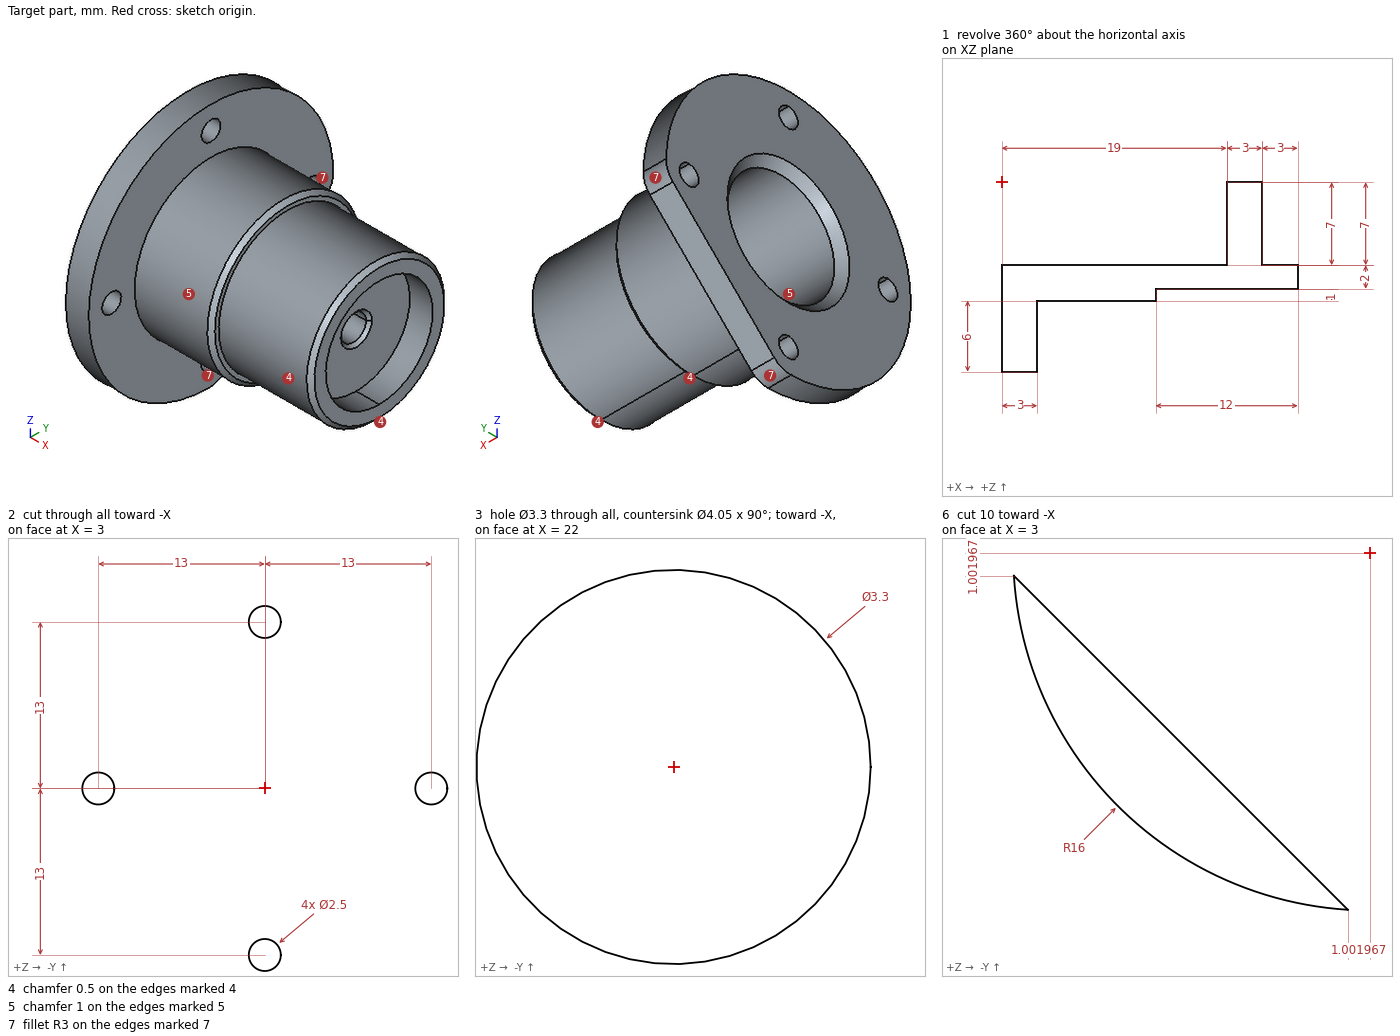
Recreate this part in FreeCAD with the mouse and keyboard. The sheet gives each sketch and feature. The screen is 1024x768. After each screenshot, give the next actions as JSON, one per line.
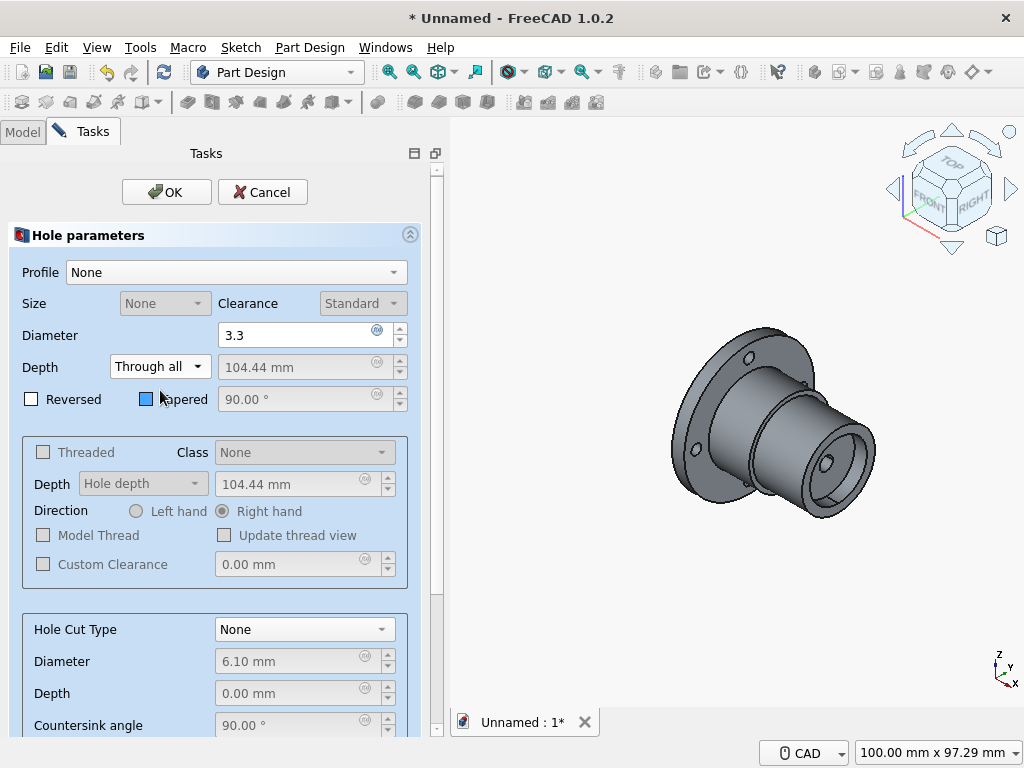
{"action": "left_click", "coordinate": [306, 630]}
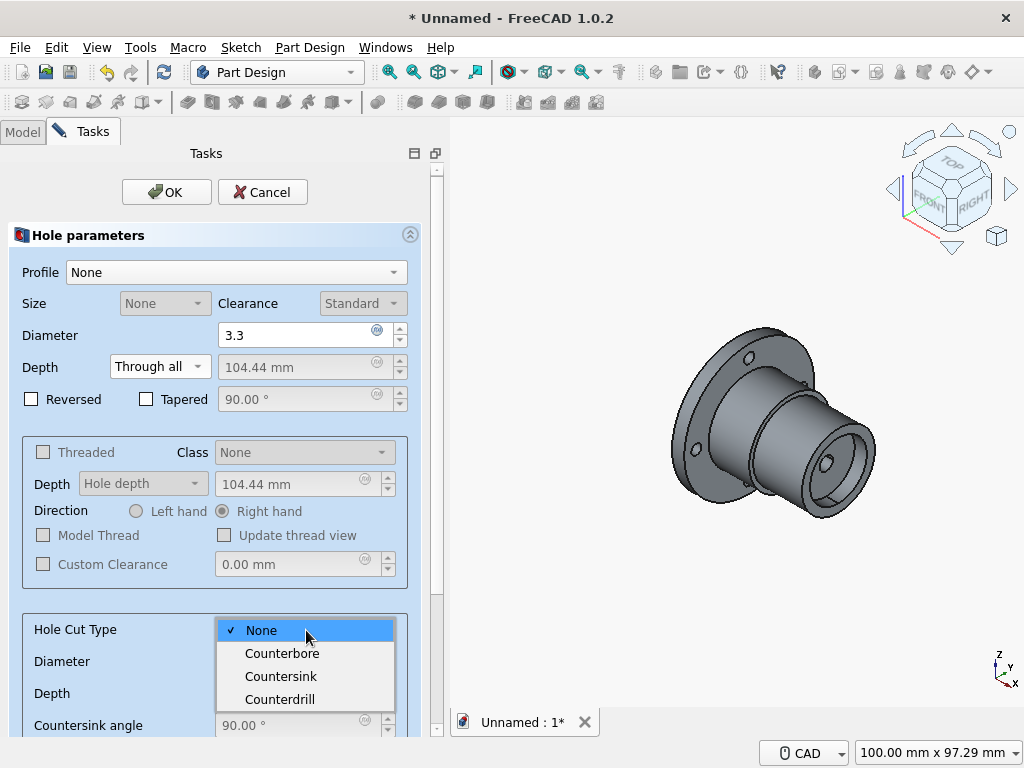
{"action": "left_click", "coordinate": [304, 676]}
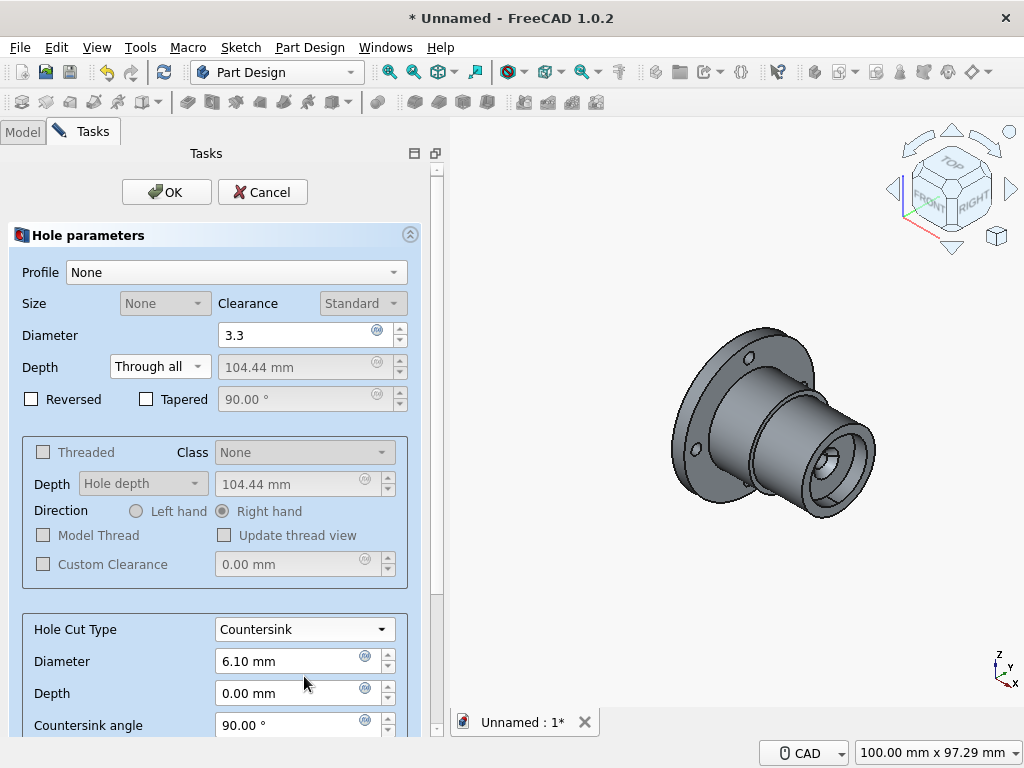
{"action": "triple_click", "coordinate": [298, 661]}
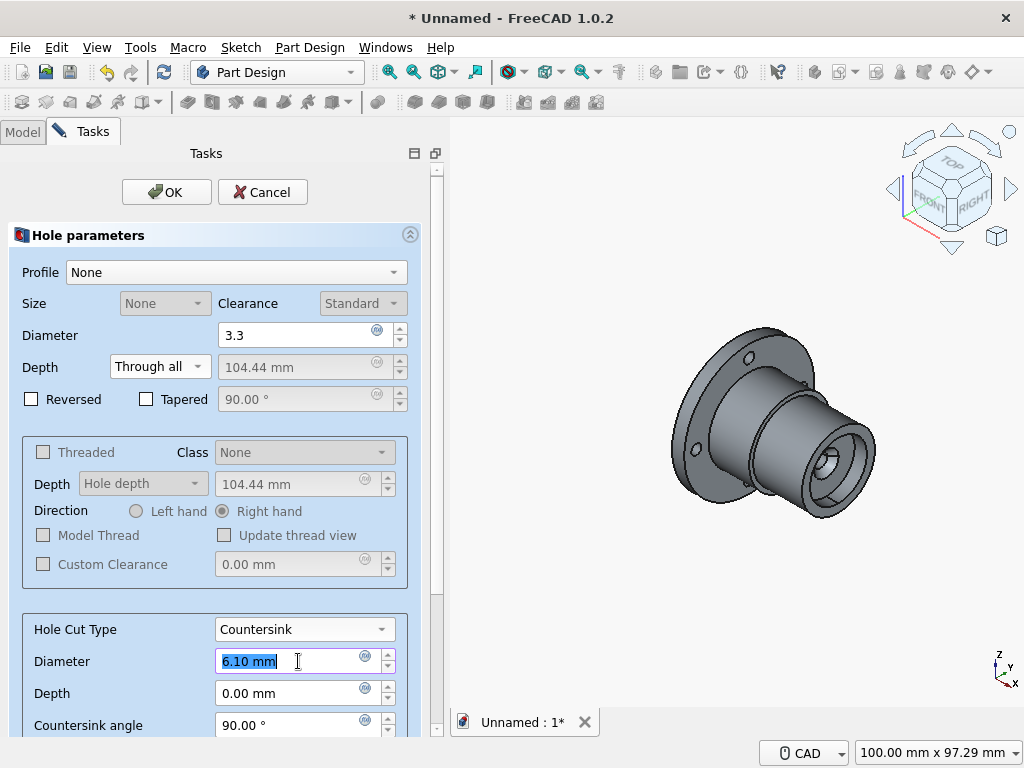
{"action": "type", "text": "4.05"}
{"action": "key", "text": "Tab"}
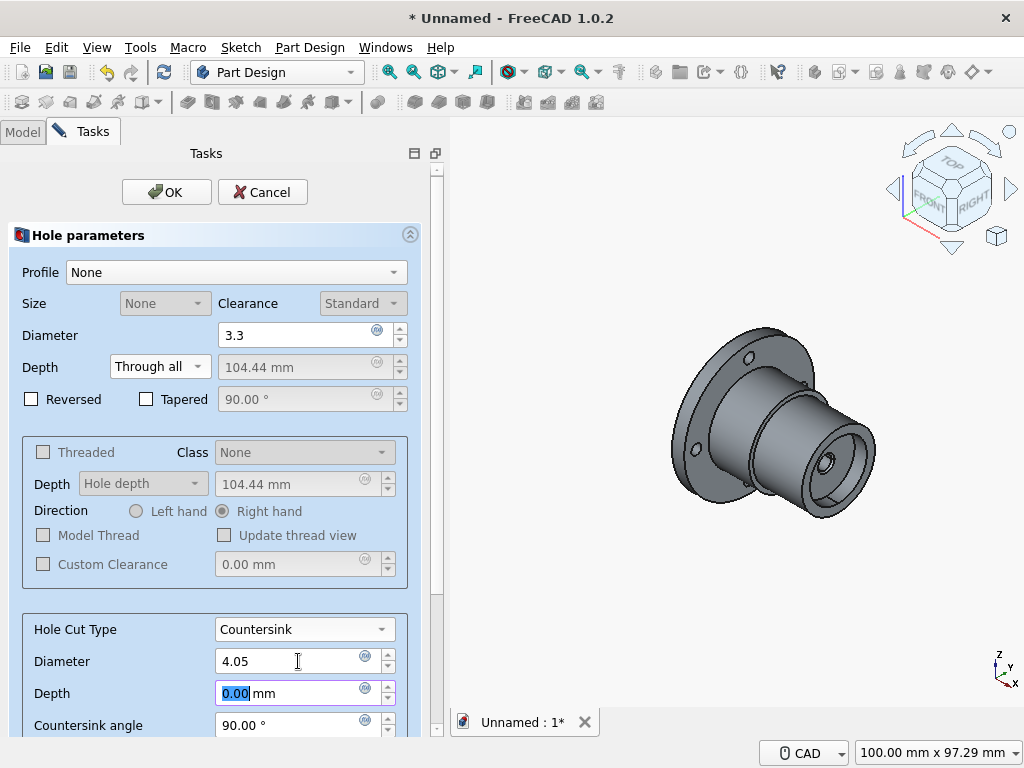
{"action": "left_click", "coordinate": [167, 192]}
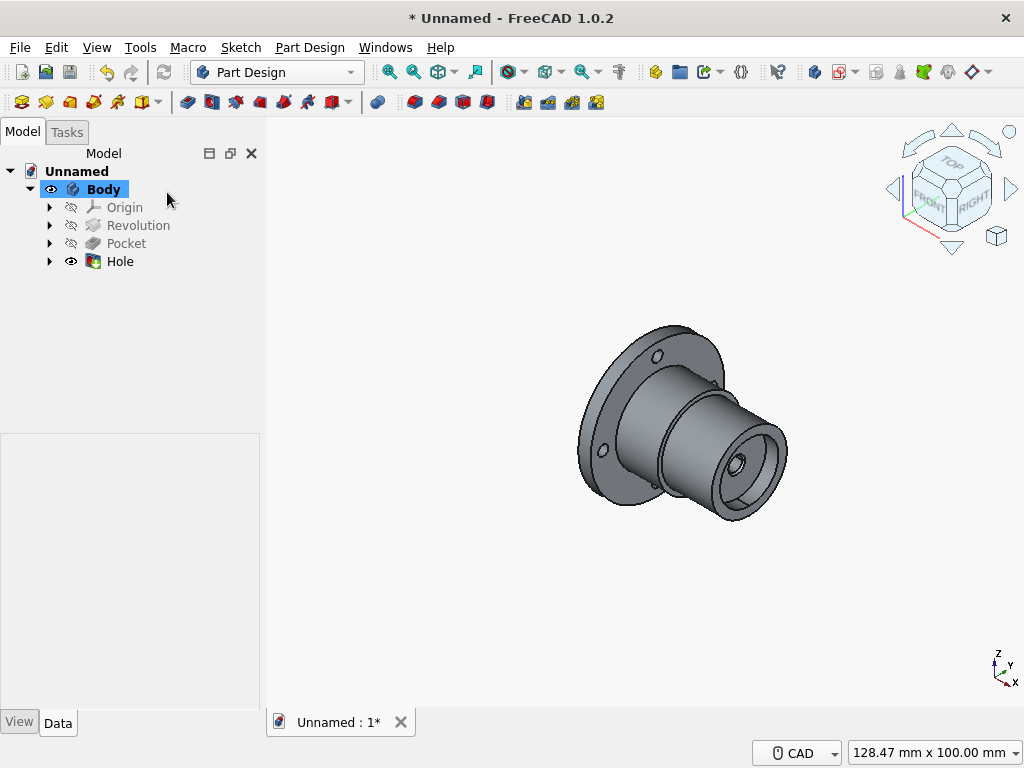
{"action": "left_click", "coordinate": [749, 428]}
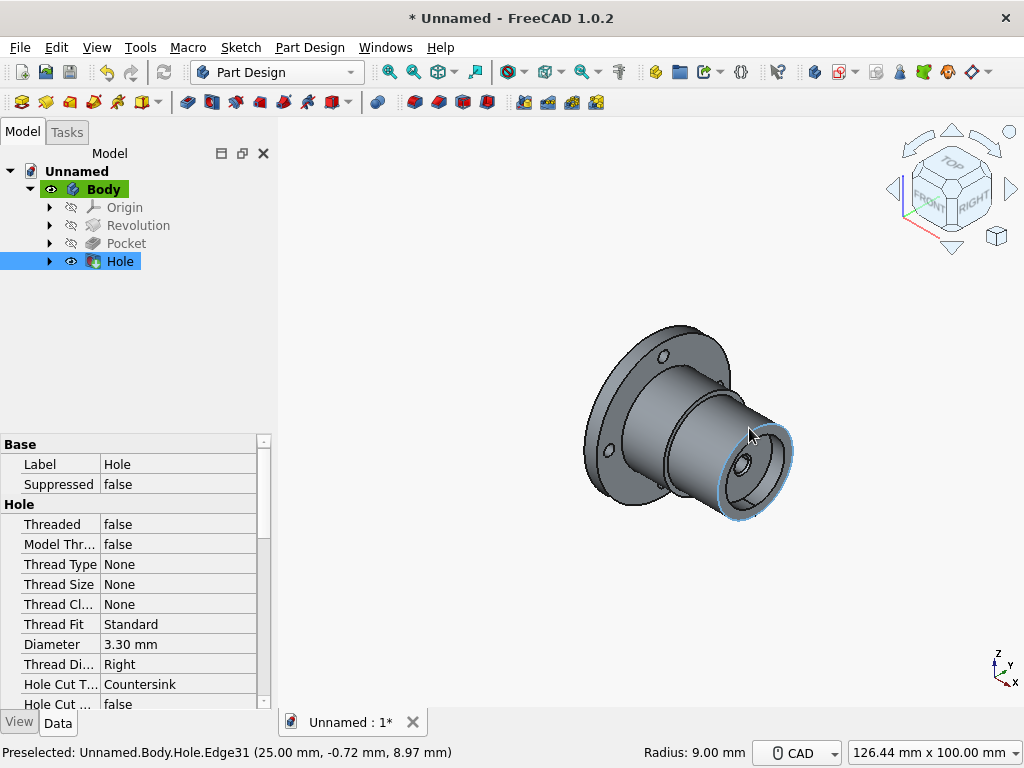
{"action": "left_click", "coordinate": [705, 394], "text": "ctrl"}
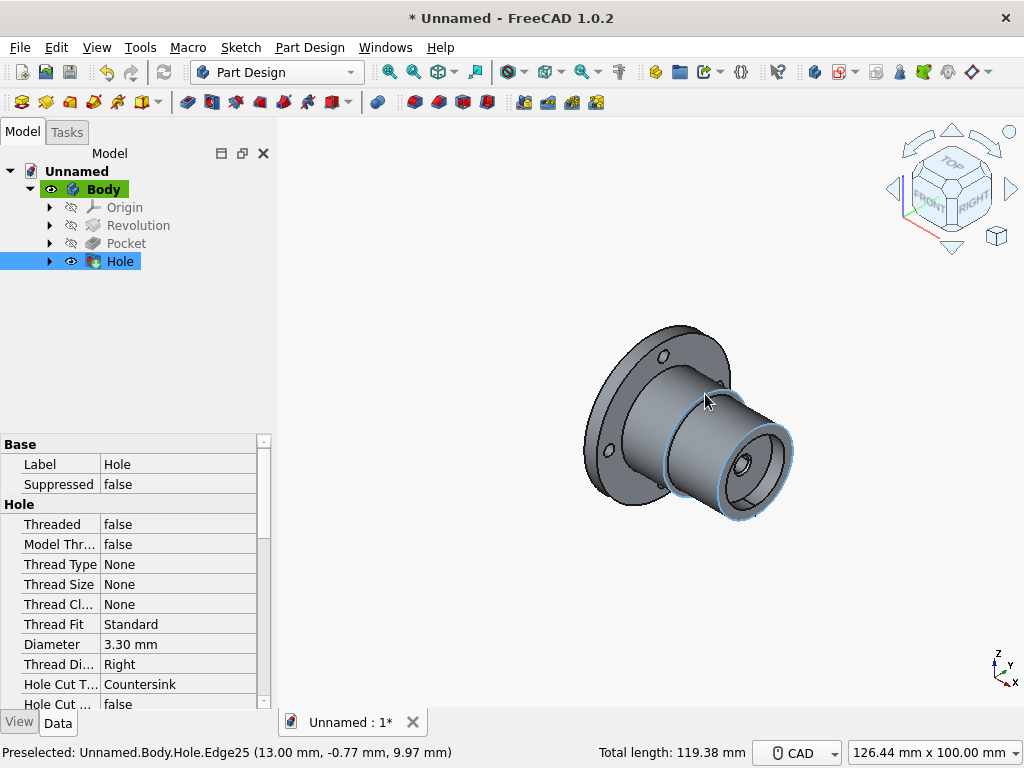
{"action": "left_click", "coordinate": [440, 102]}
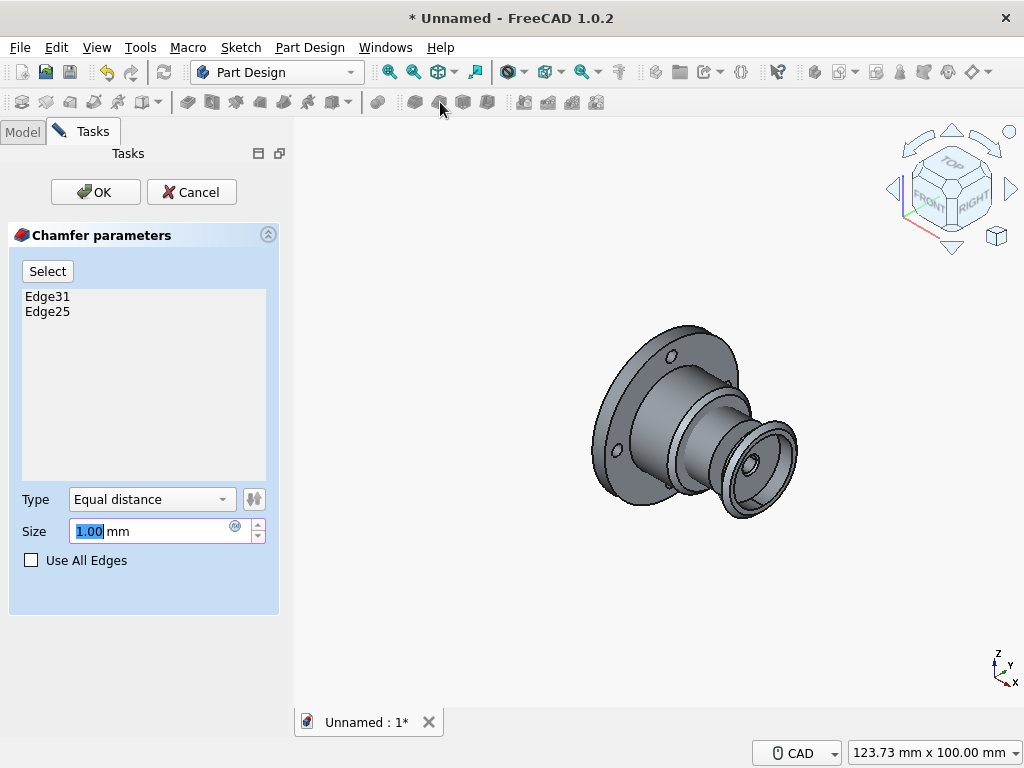
{"action": "type", "text": "0.5"}
{"action": "key", "text": "Tab"}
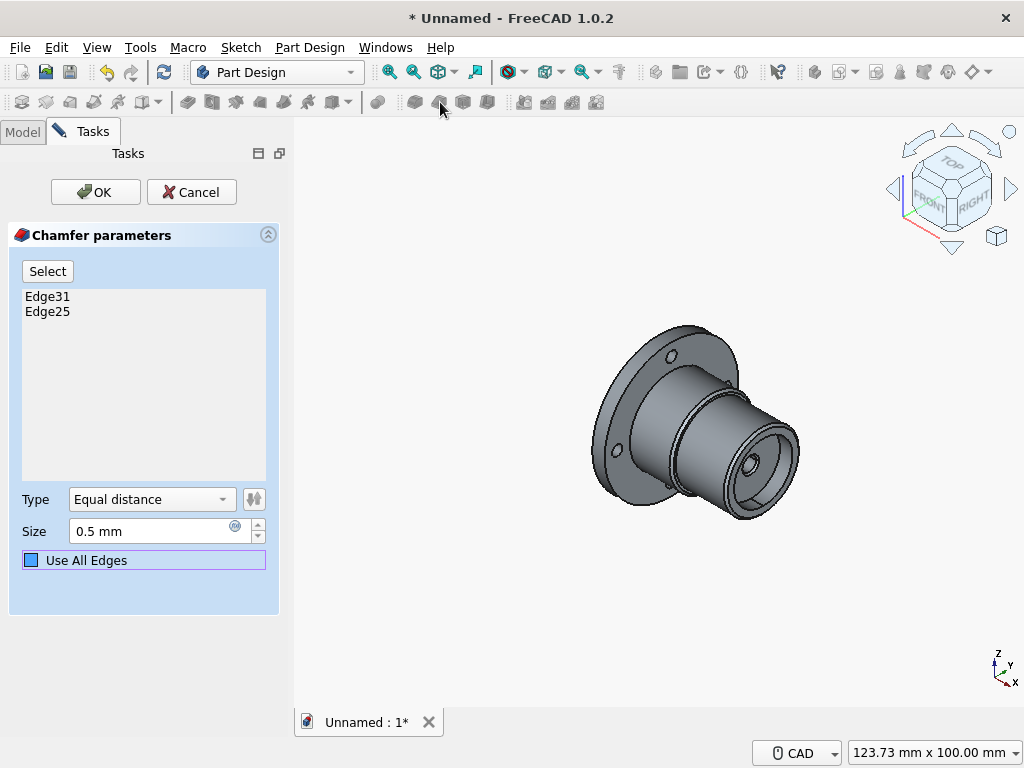
{"action": "left_click", "coordinate": [96, 192]}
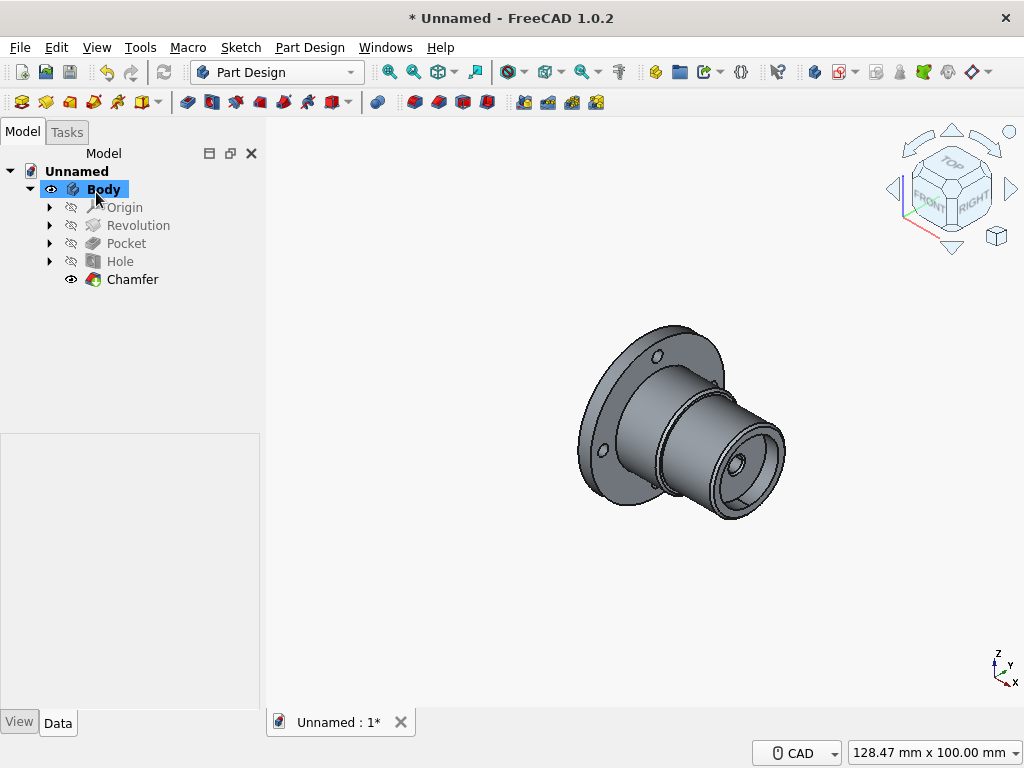
{"action": "key", "text": "2"}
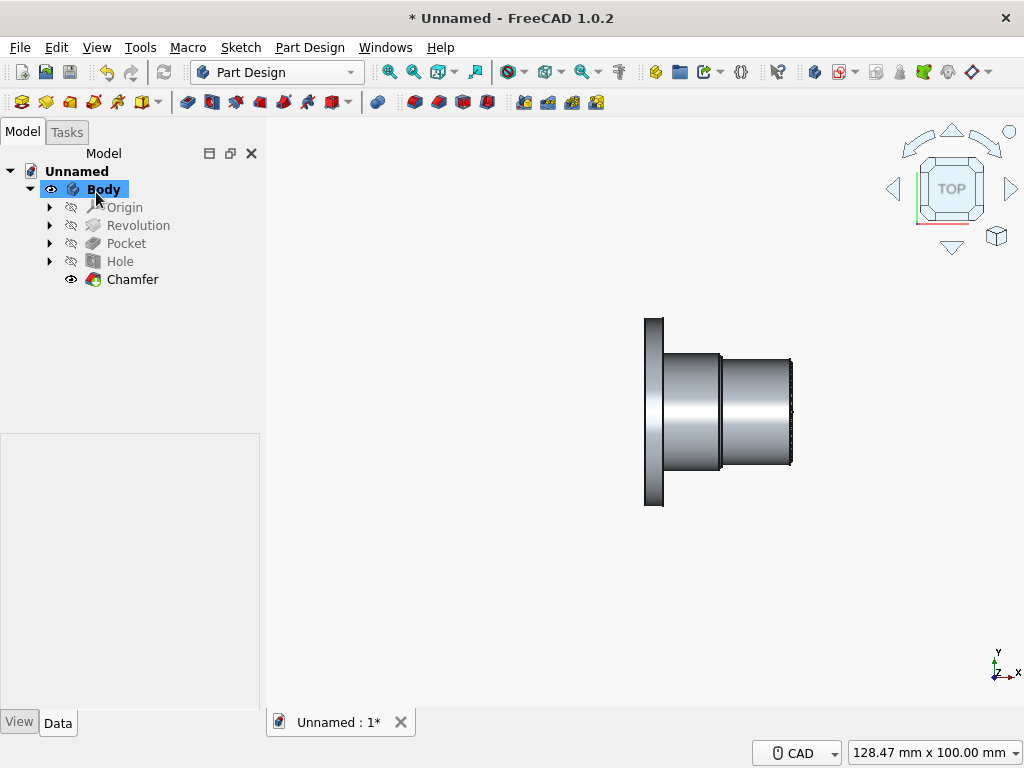
{"action": "left_click", "coordinate": [390, 72]}